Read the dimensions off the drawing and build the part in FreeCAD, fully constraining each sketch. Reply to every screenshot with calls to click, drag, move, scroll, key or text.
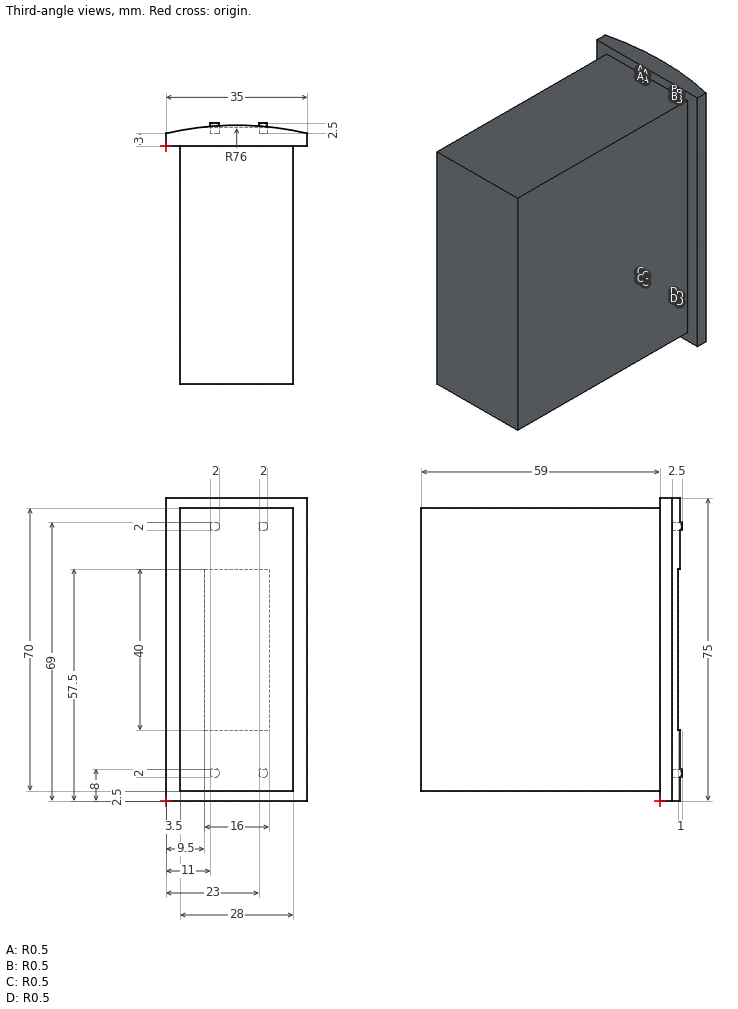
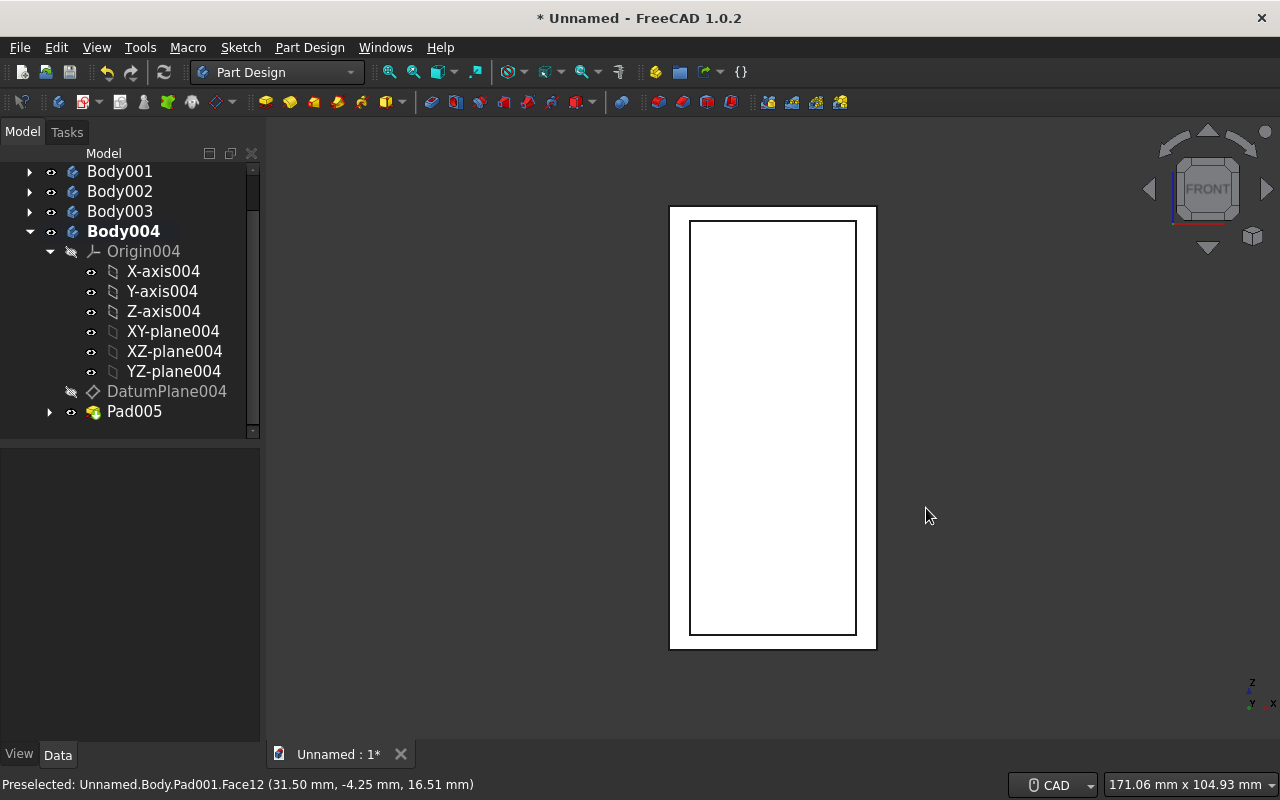
scroll(806, 602, up, 5)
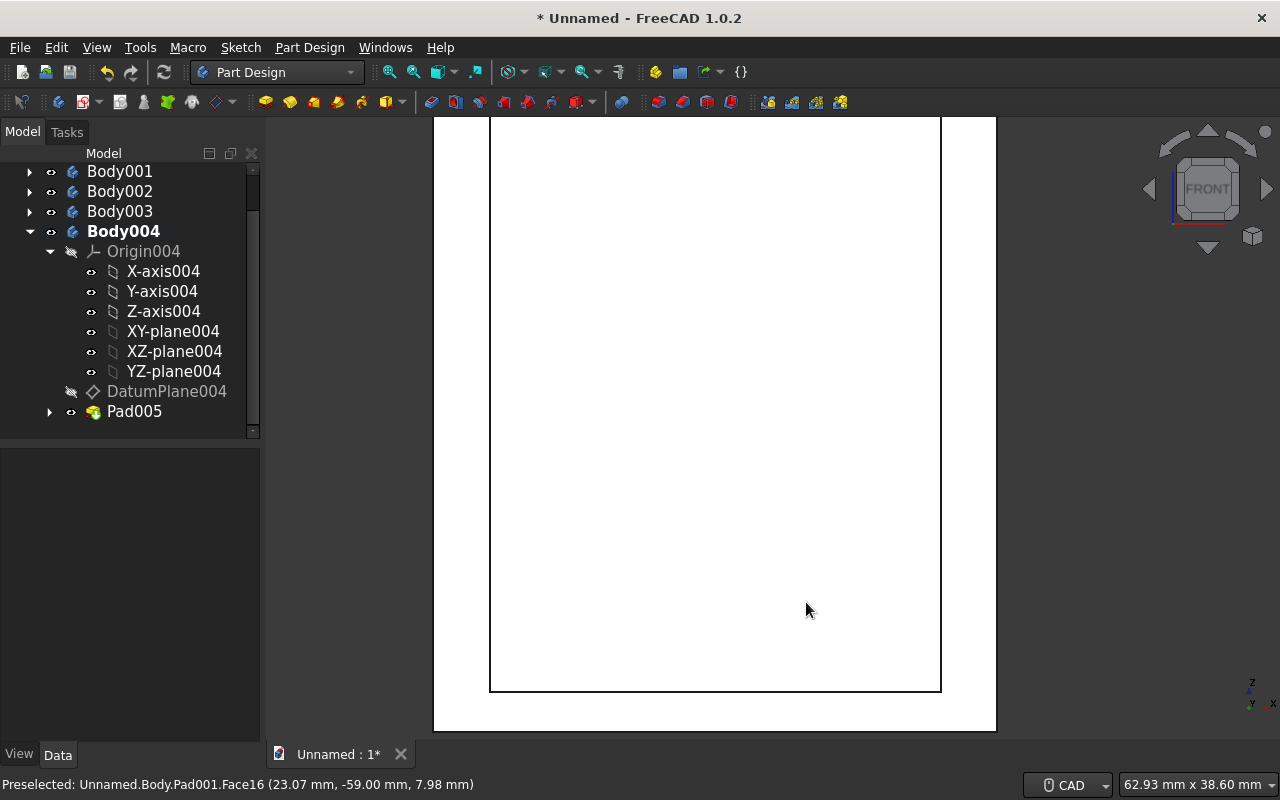
key(v)
key(f)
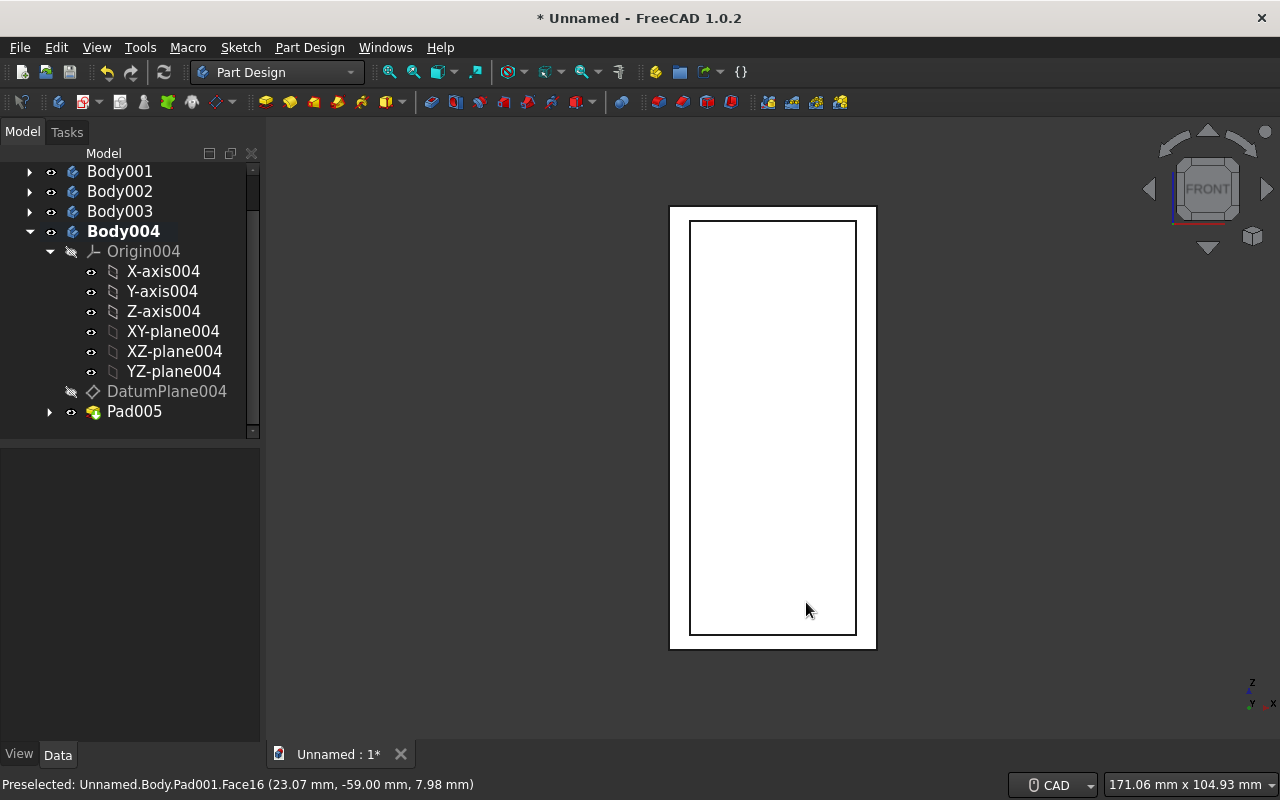
key(3)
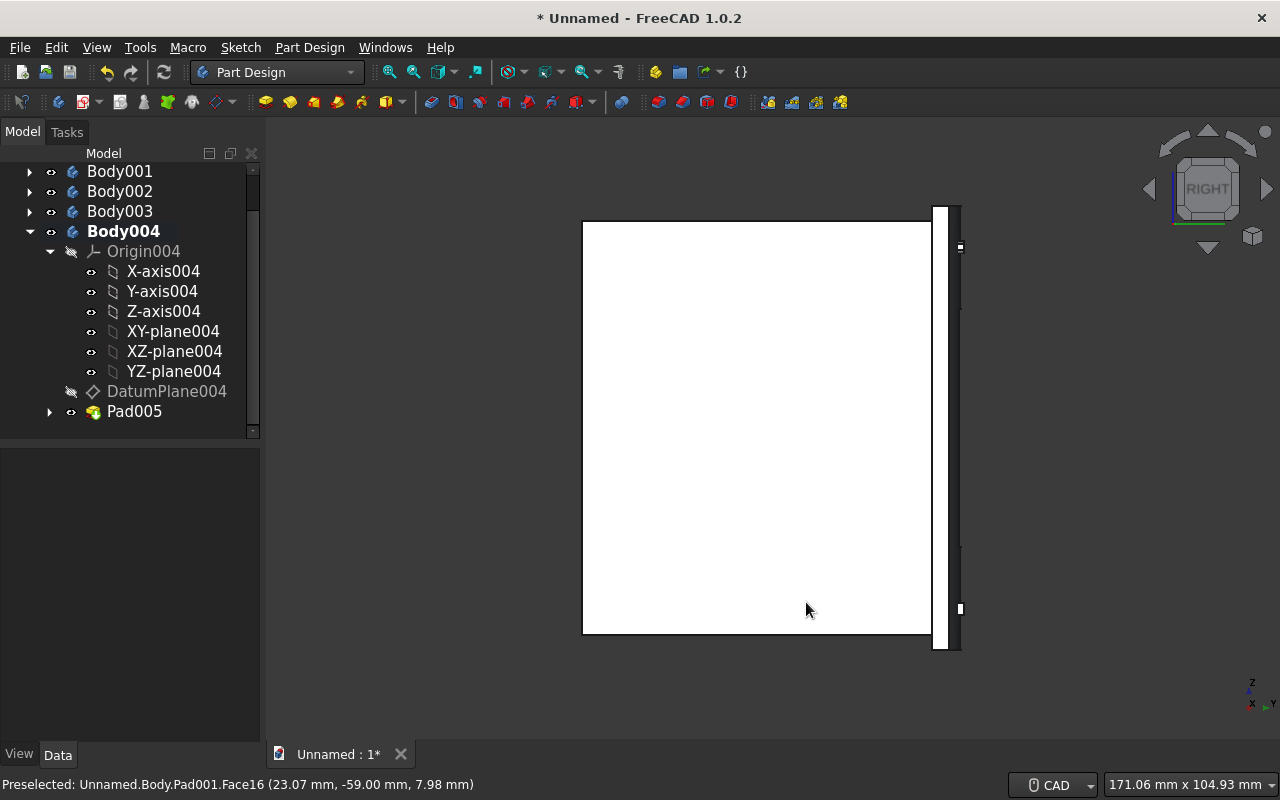
key(v)
key(f)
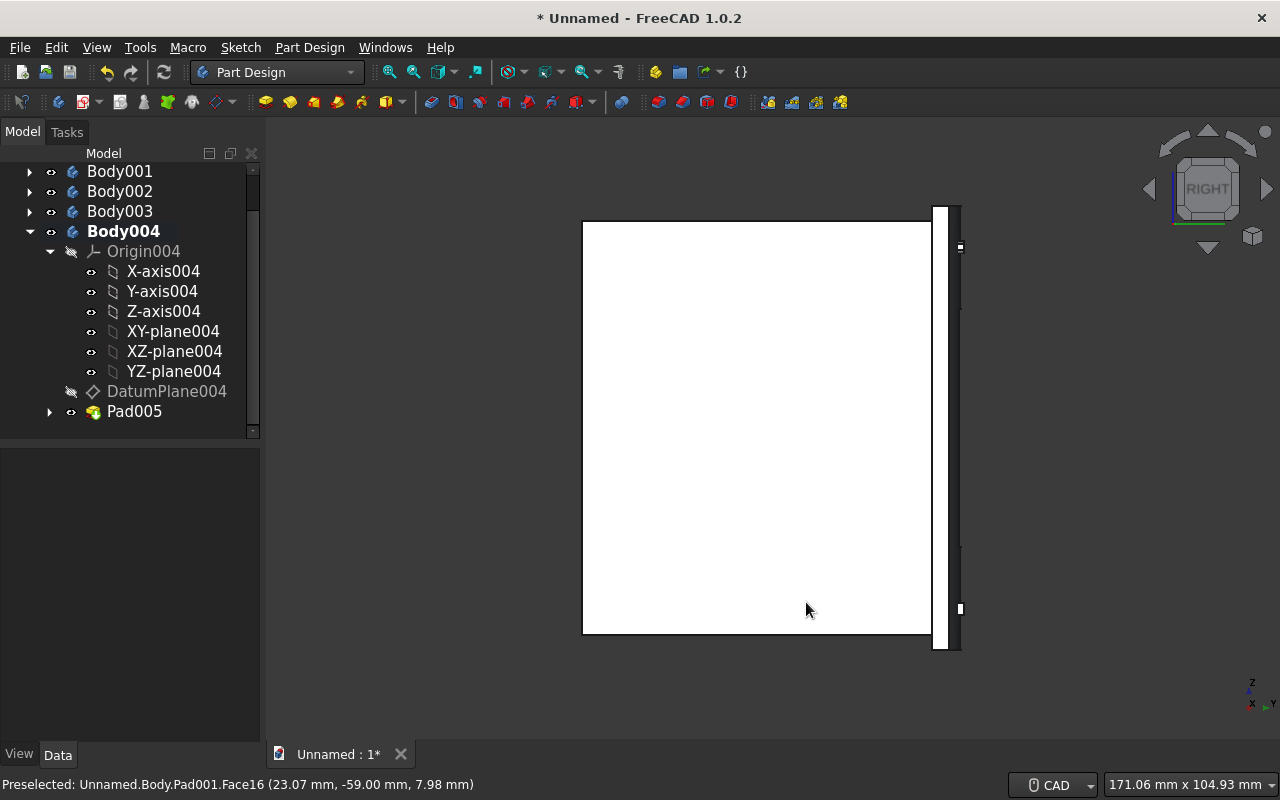
scroll(957, 602, up, 5)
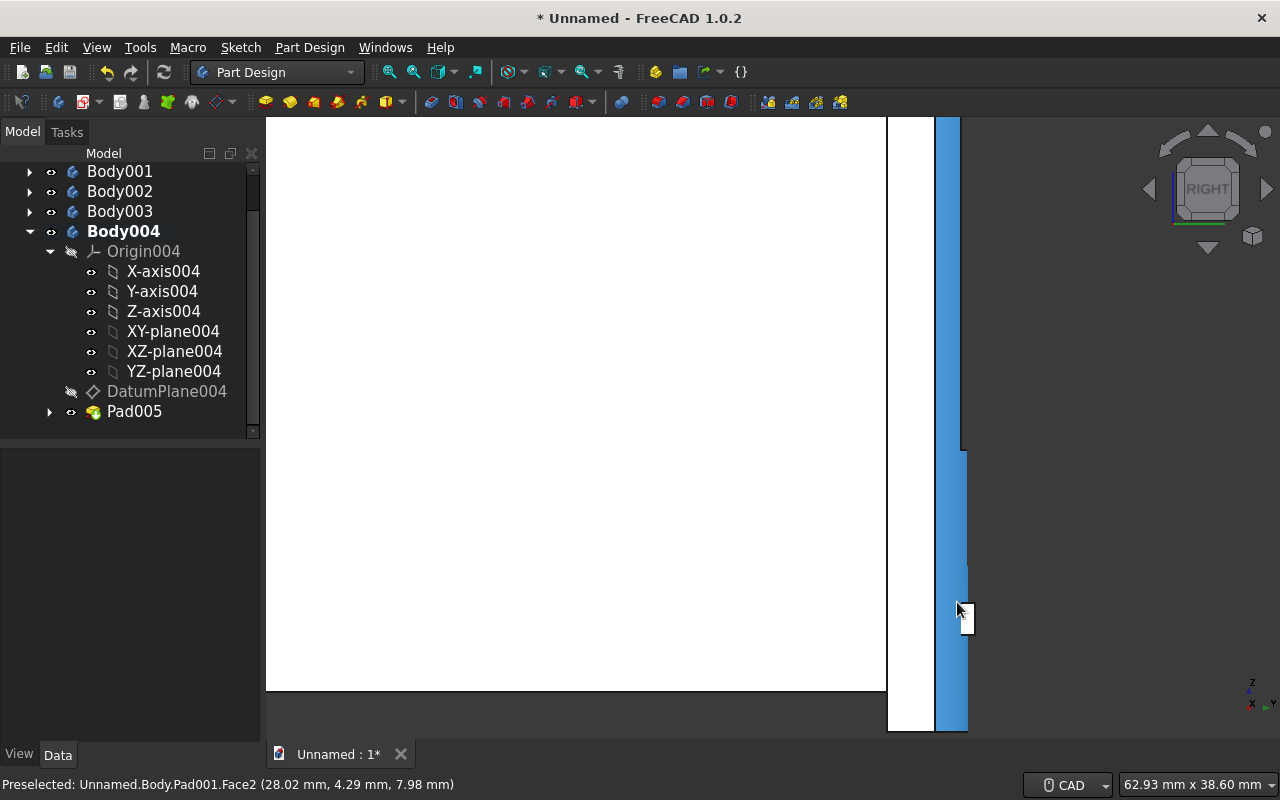
click(963, 602)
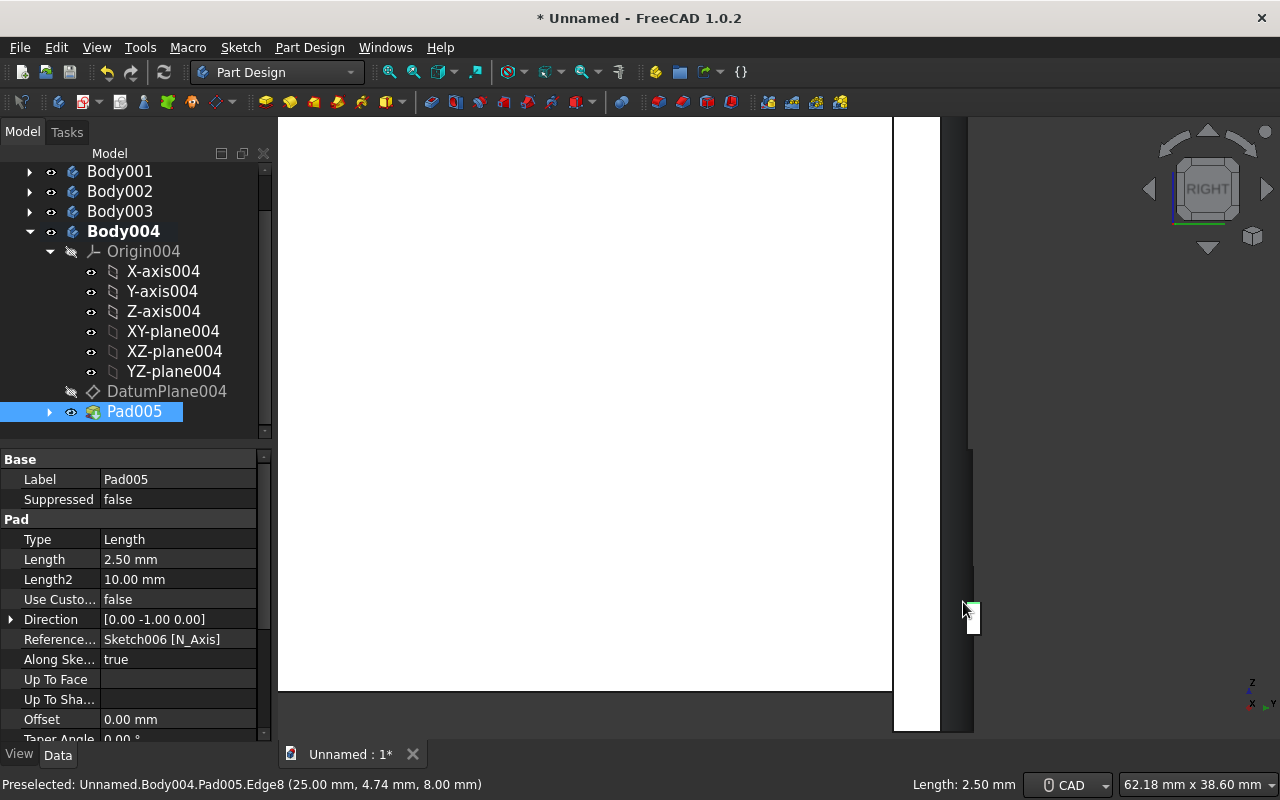
key(v)
key(f)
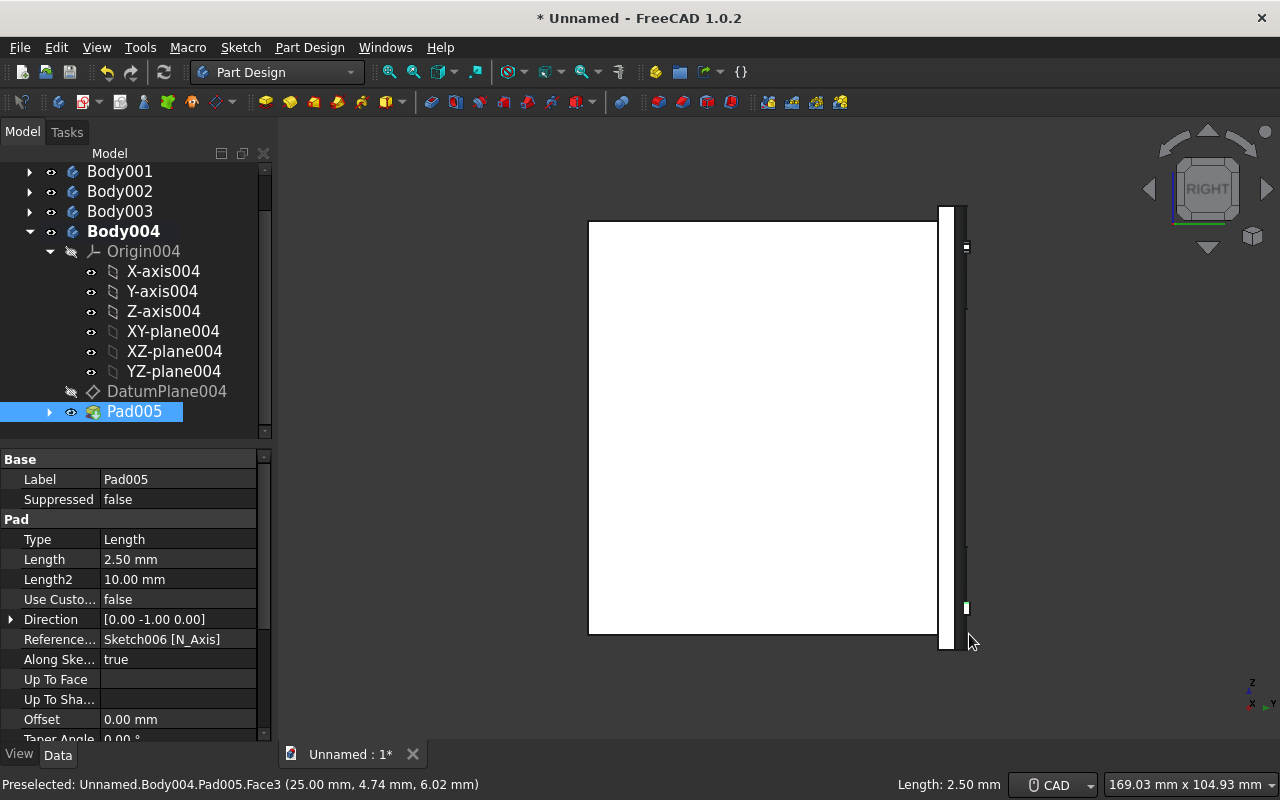
key(5)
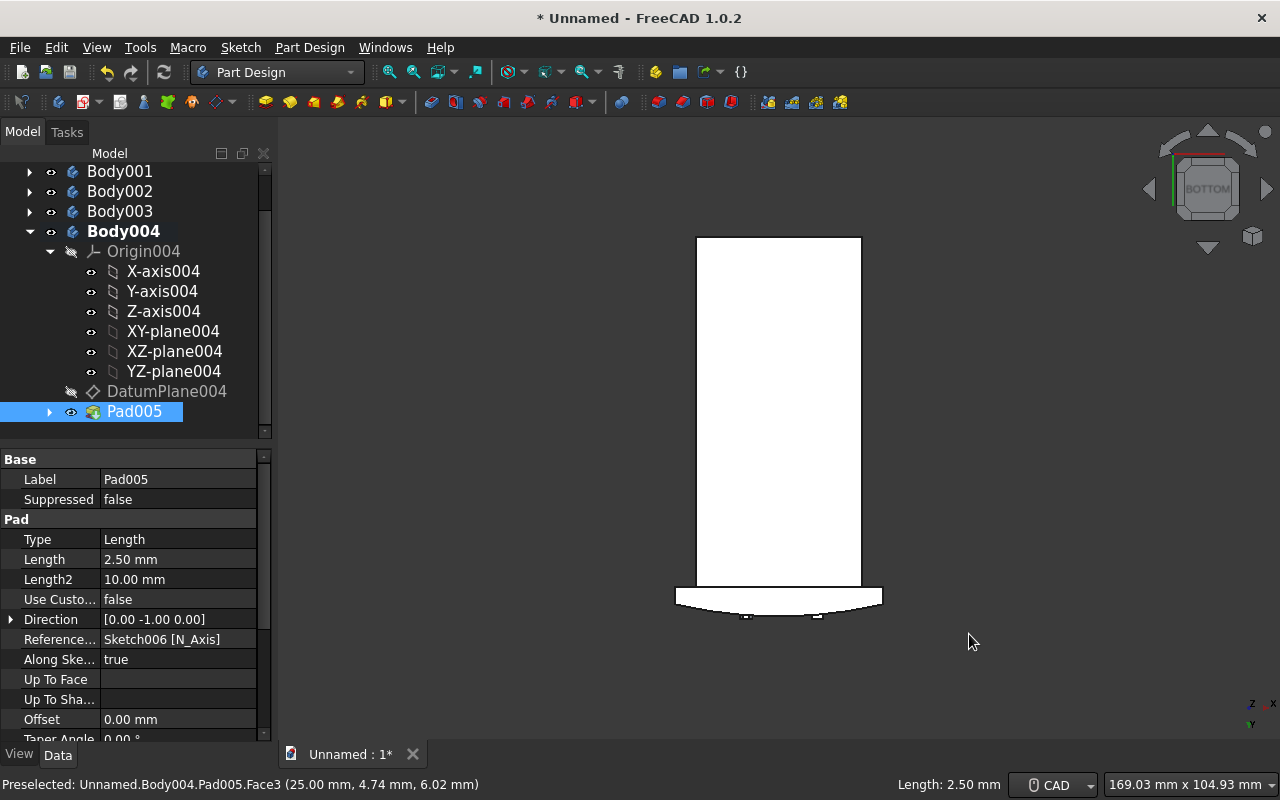
click(390, 72)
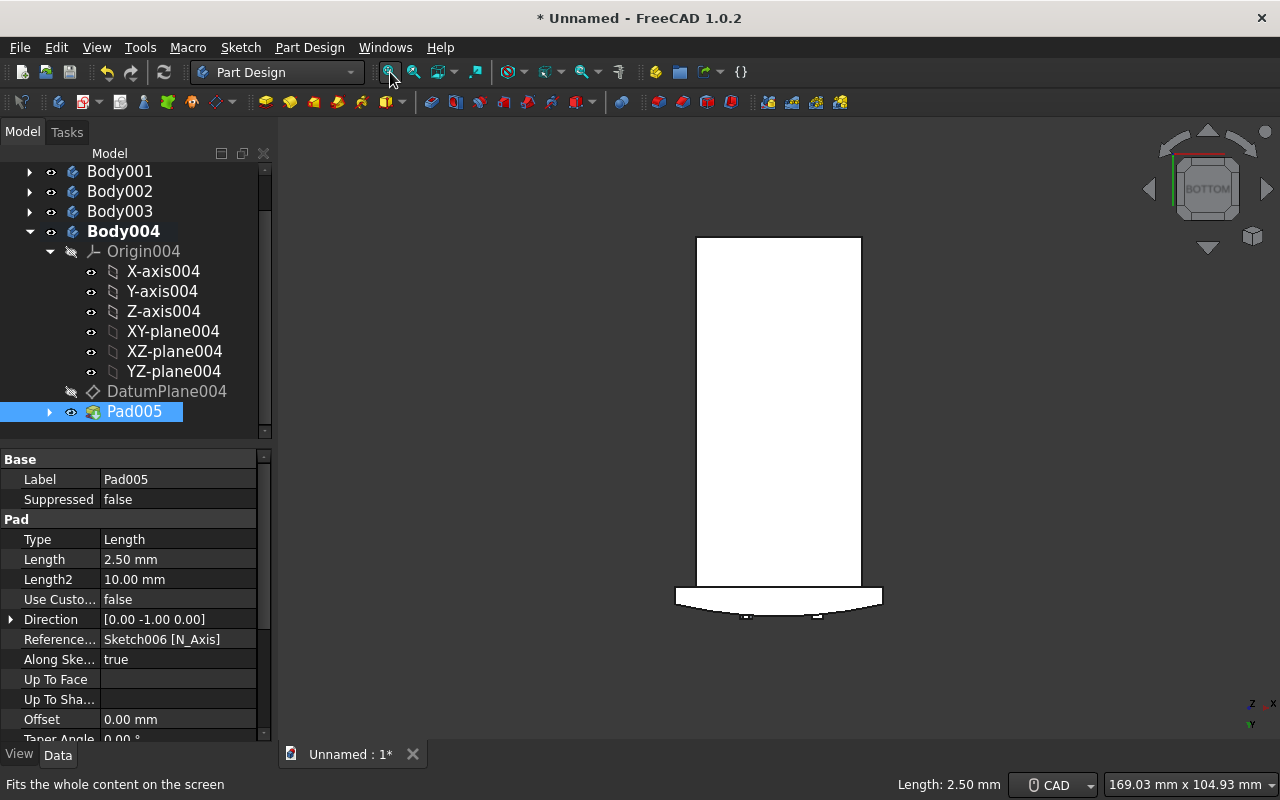
scroll(812, 611, up, 5)